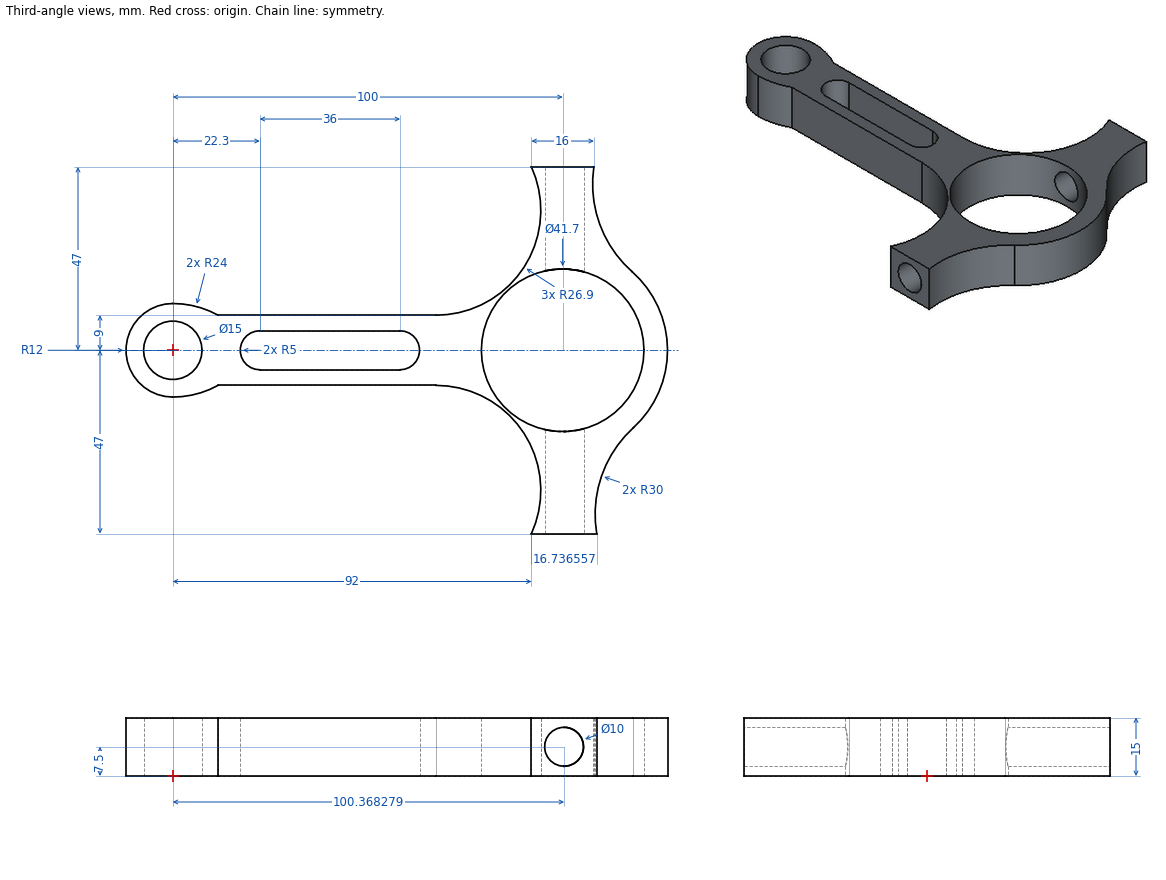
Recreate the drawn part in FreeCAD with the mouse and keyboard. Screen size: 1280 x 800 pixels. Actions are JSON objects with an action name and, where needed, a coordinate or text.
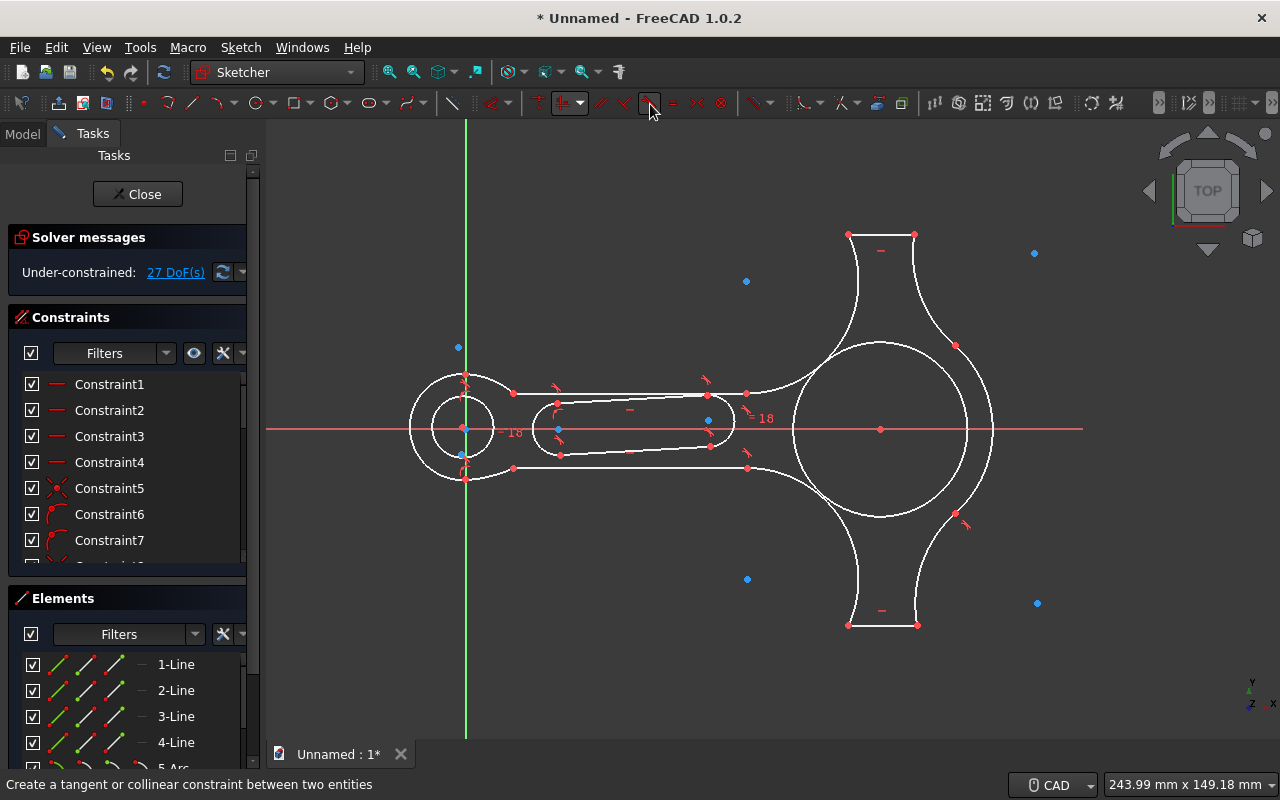
{"action": "left_click", "coordinate": [987, 466]}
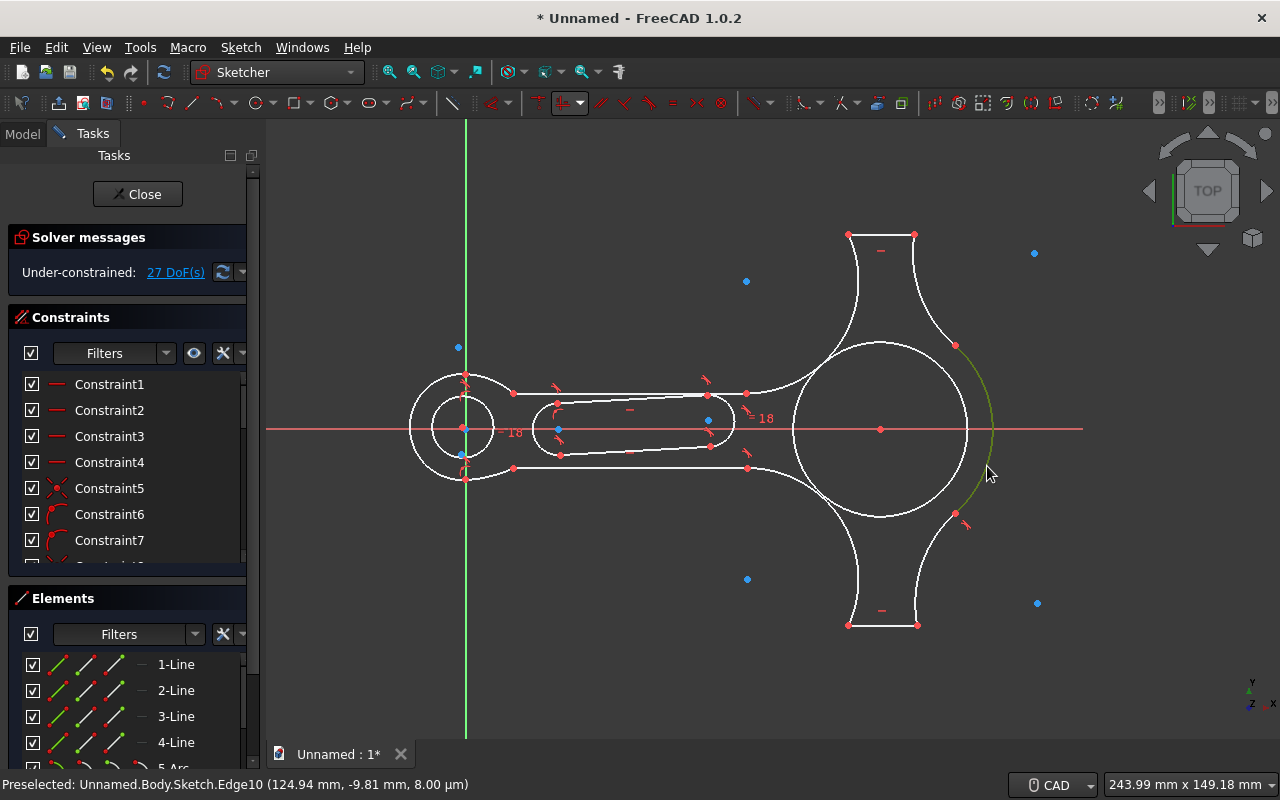
{"action": "left_click", "coordinate": [914, 272]}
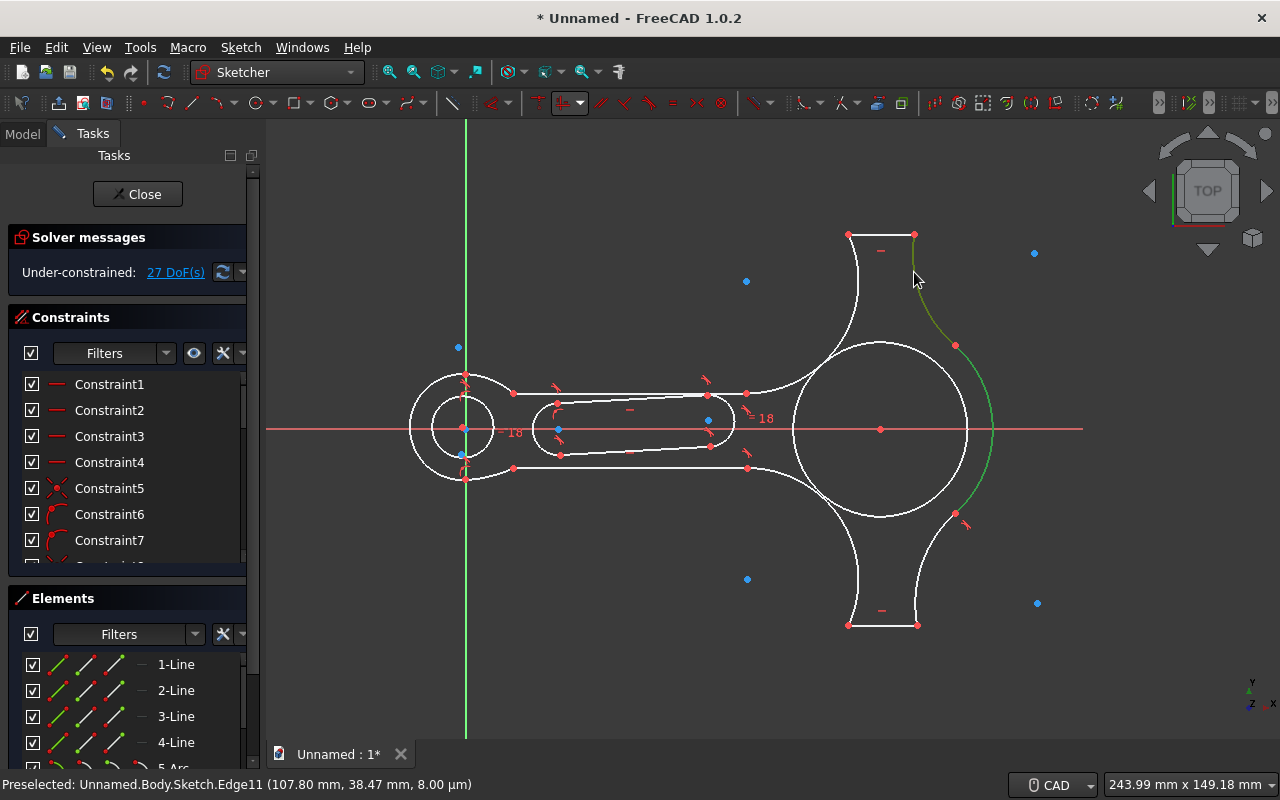
{"action": "left_click", "coordinate": [650, 104]}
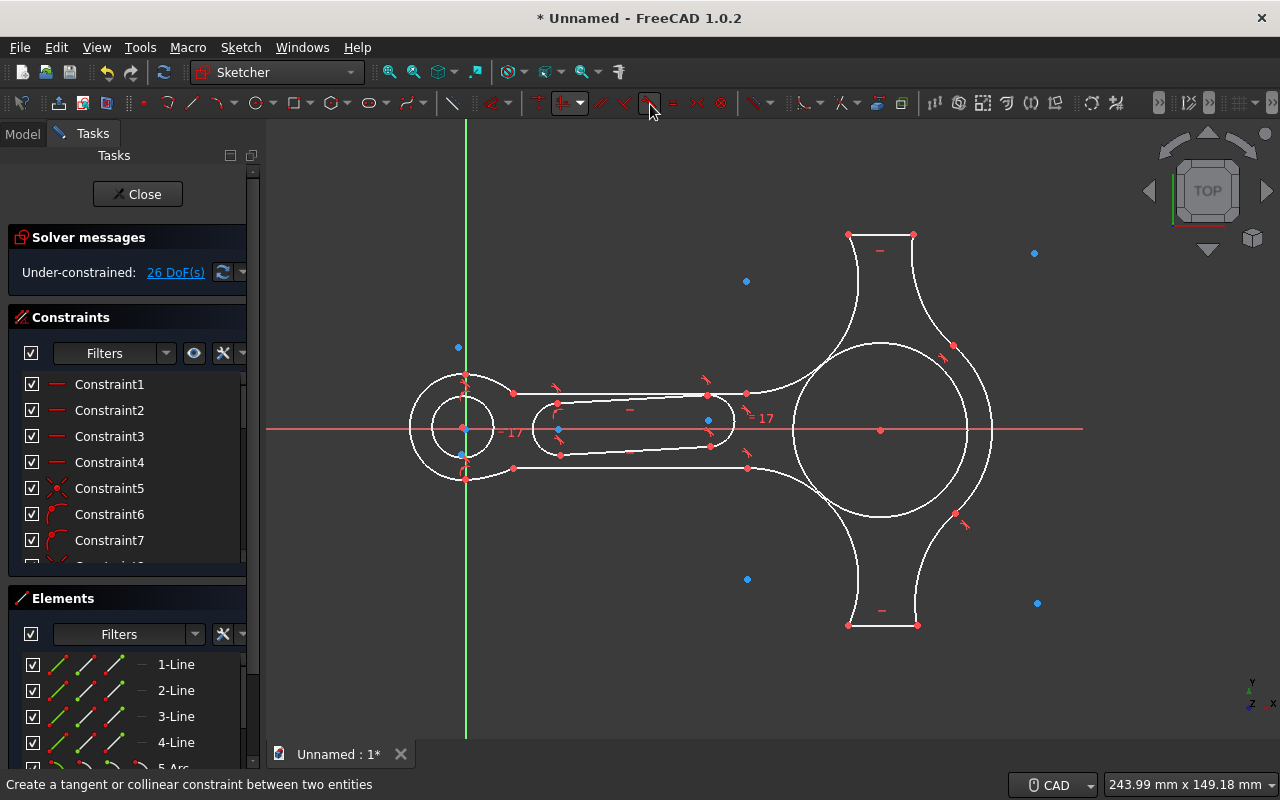
{"action": "scroll", "coordinate": [587, 402], "scroll_direction": "up", "scroll_amount": 3}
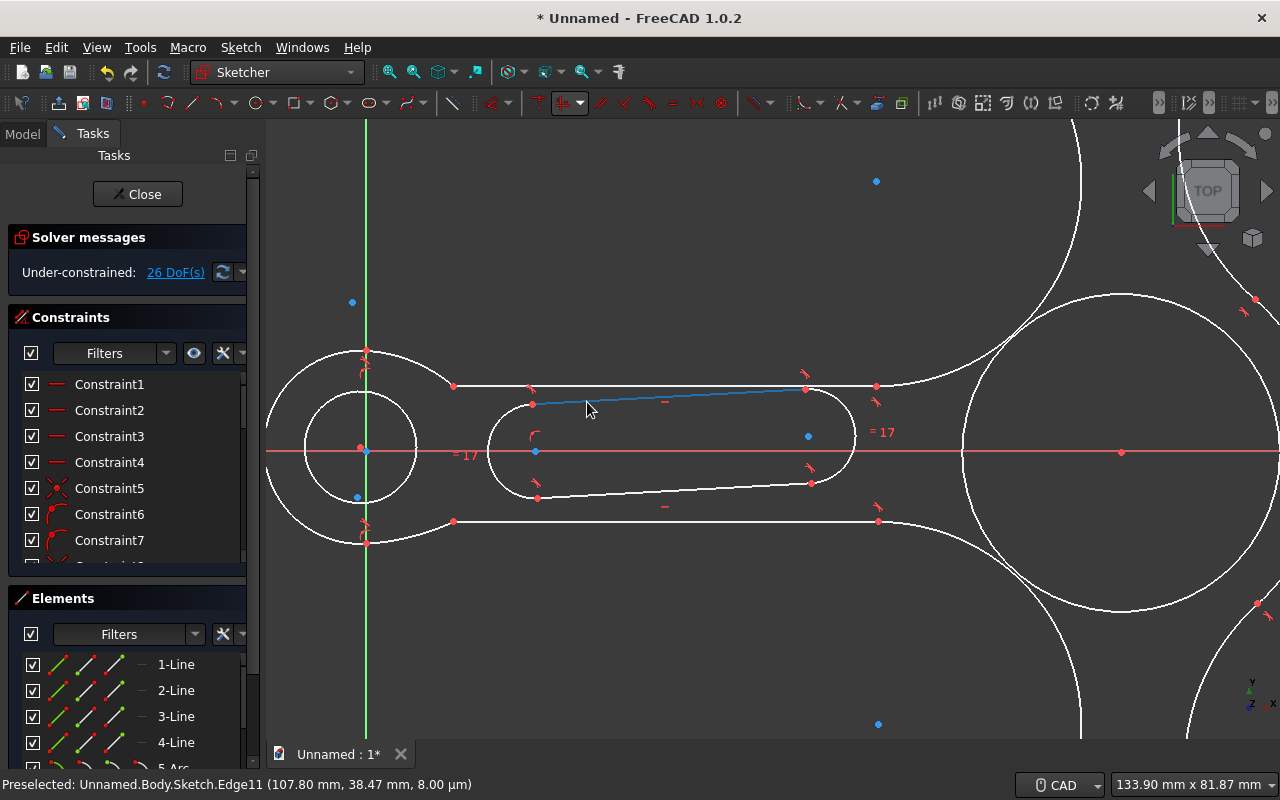
{"action": "left_click", "coordinate": [587, 401]}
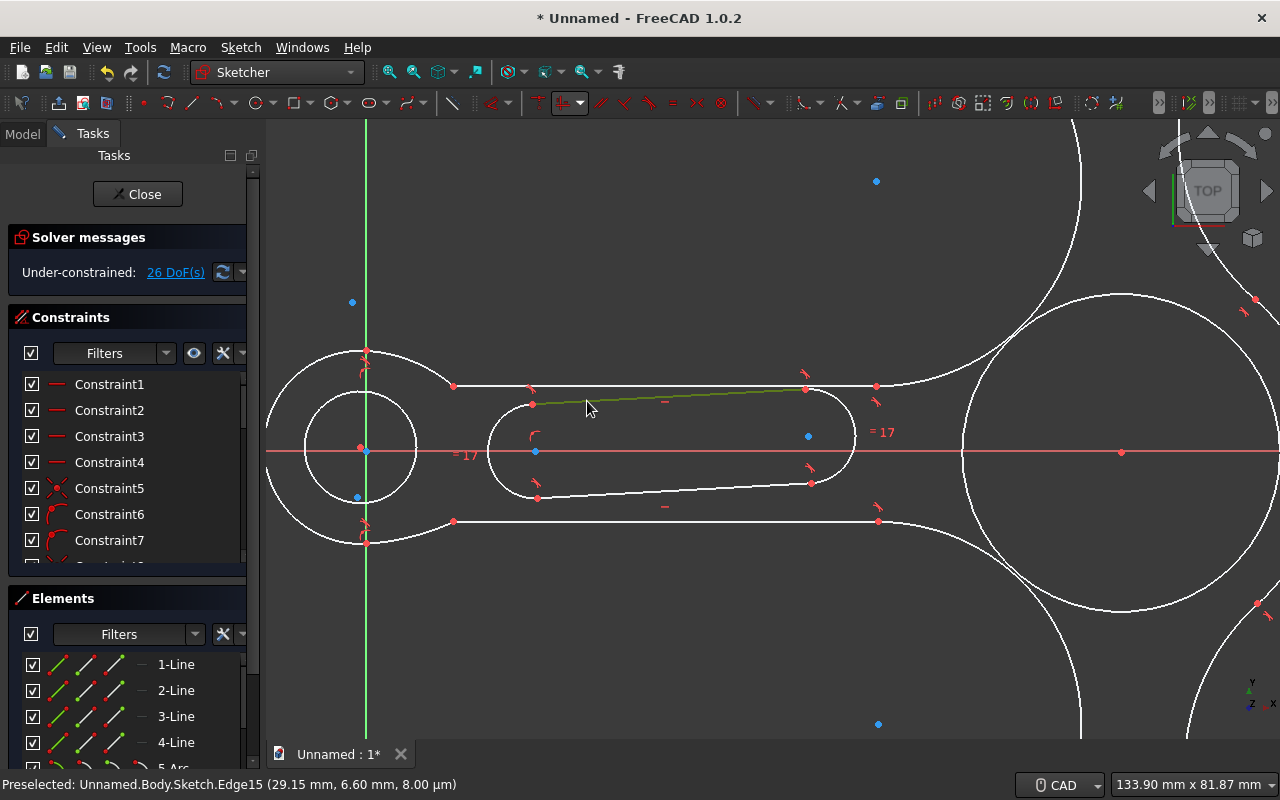
{"action": "key", "text": "h"}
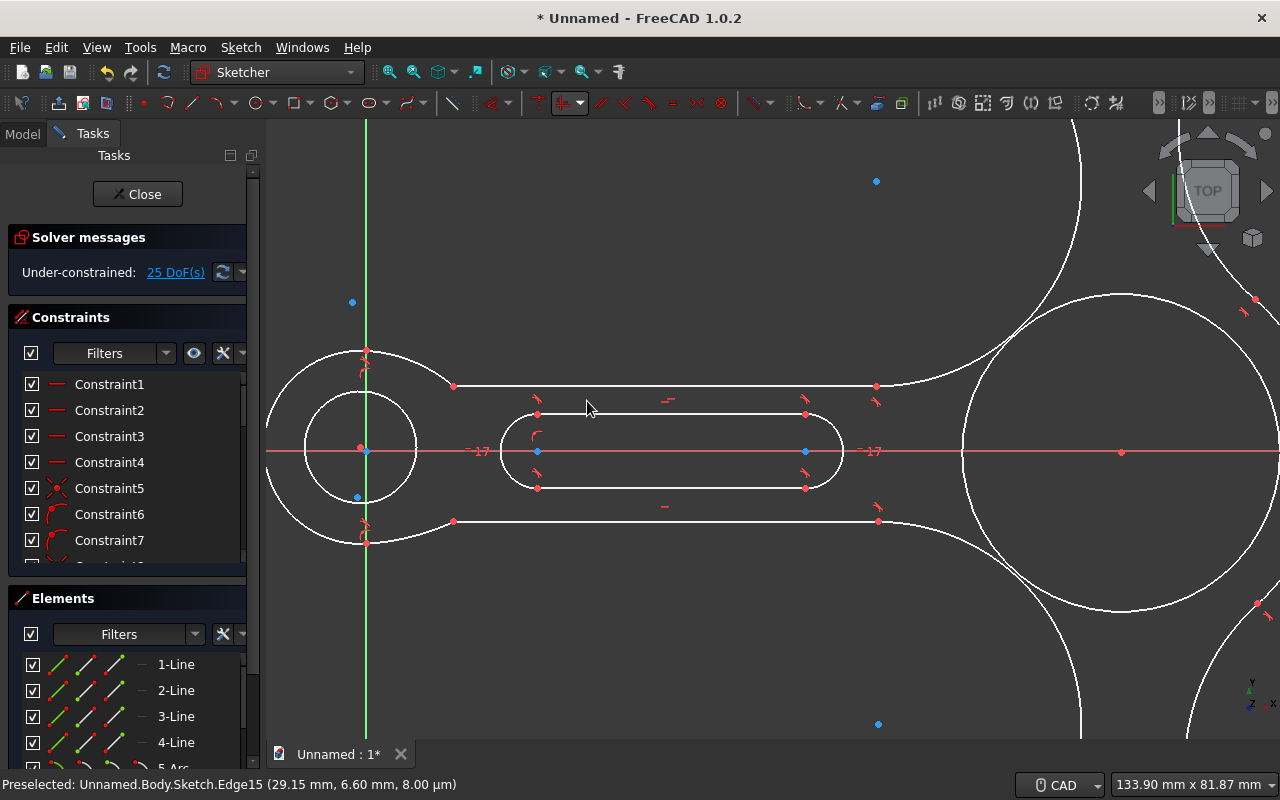
{"action": "left_click_drag", "start_coordinate": [351, 437], "coordinate": [376, 461]}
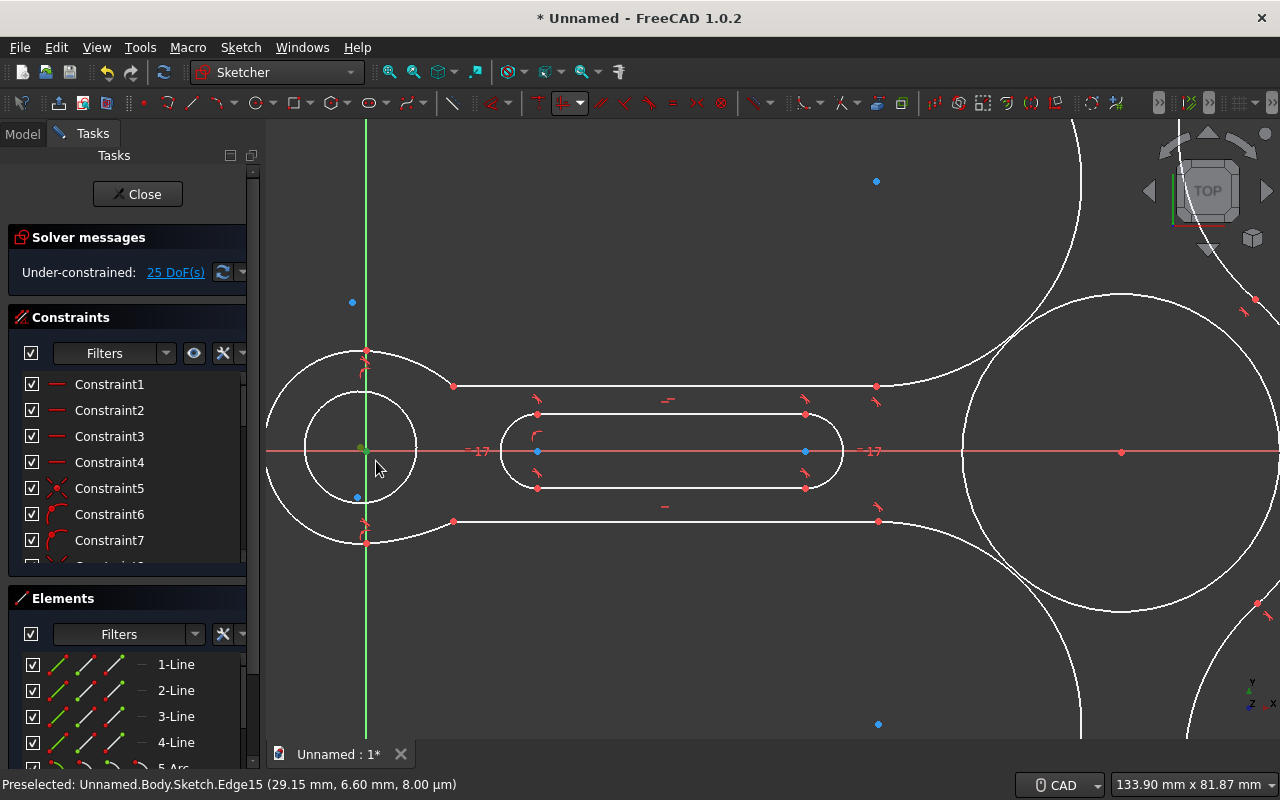
{"action": "left_click", "coordinate": [538, 104]}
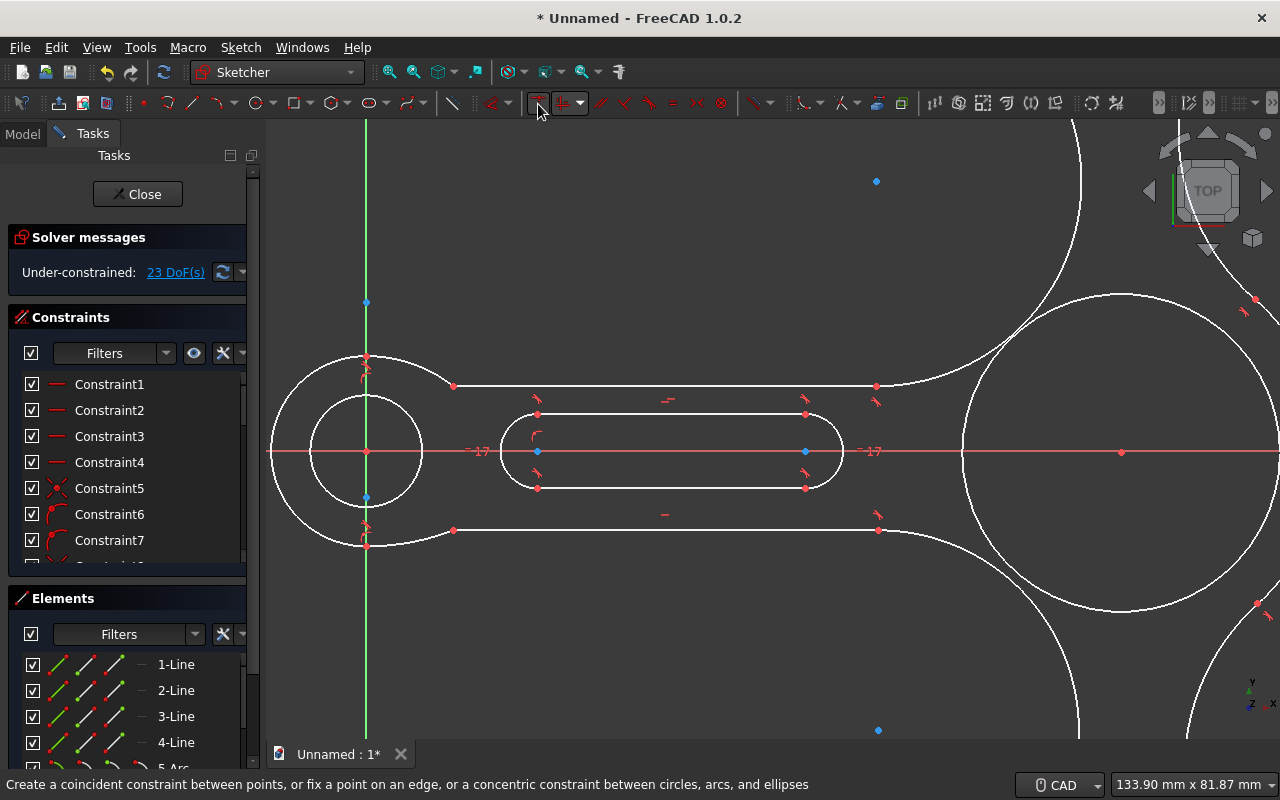
{"action": "left_click", "coordinate": [430, 371]}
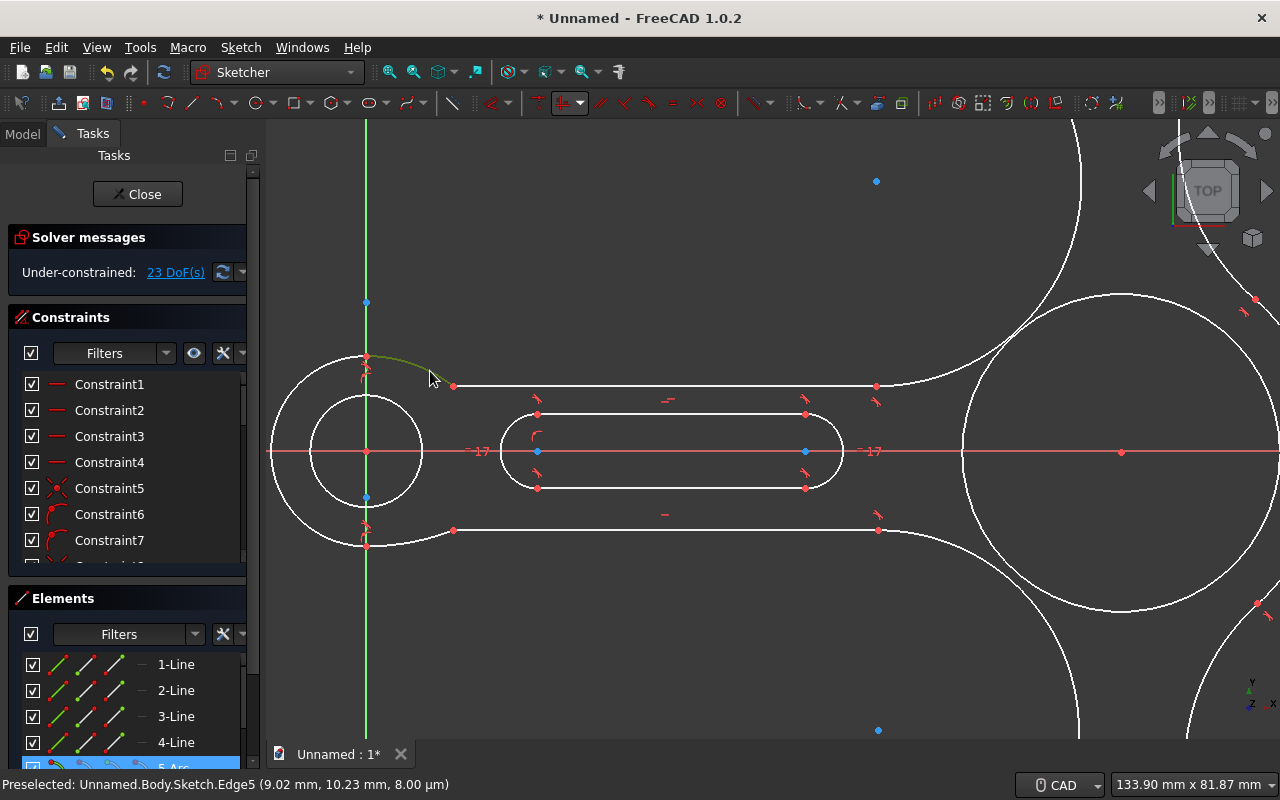
{"action": "left_click", "coordinate": [393, 545]}